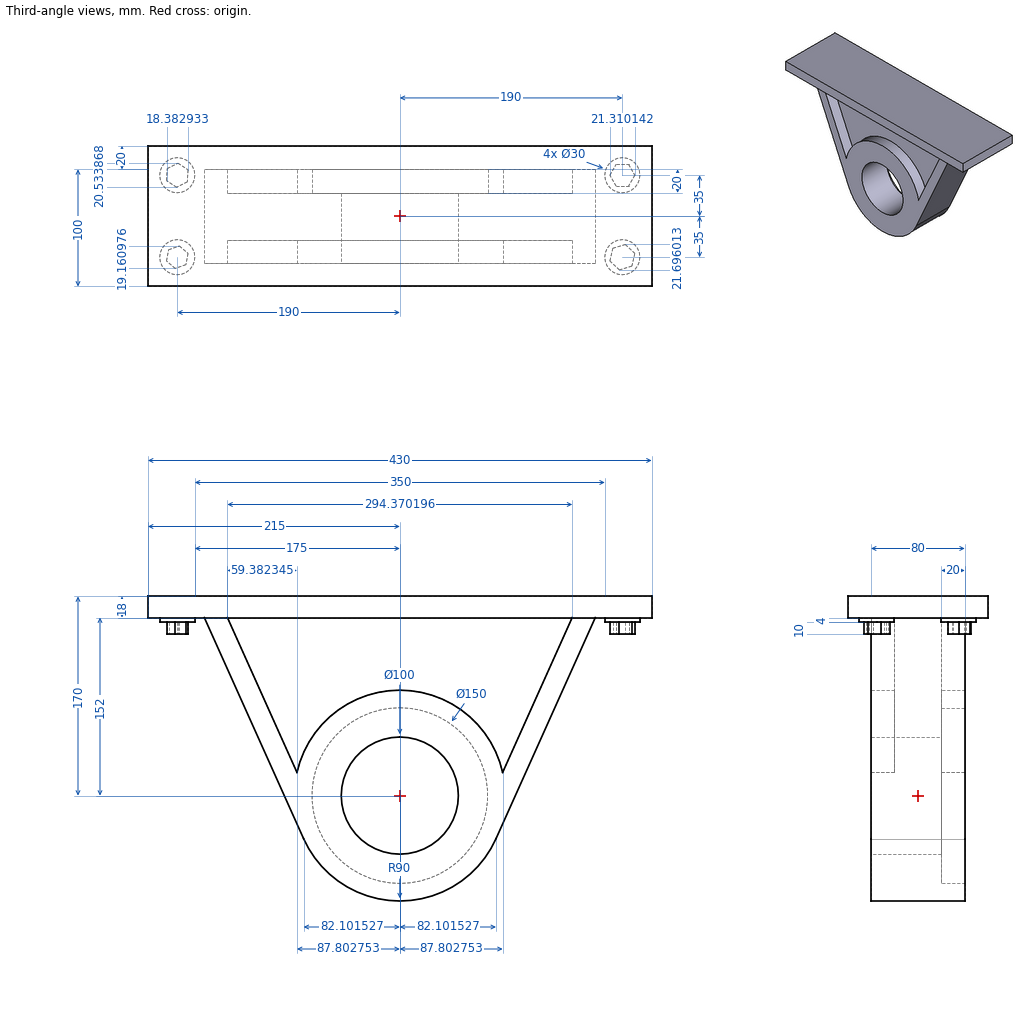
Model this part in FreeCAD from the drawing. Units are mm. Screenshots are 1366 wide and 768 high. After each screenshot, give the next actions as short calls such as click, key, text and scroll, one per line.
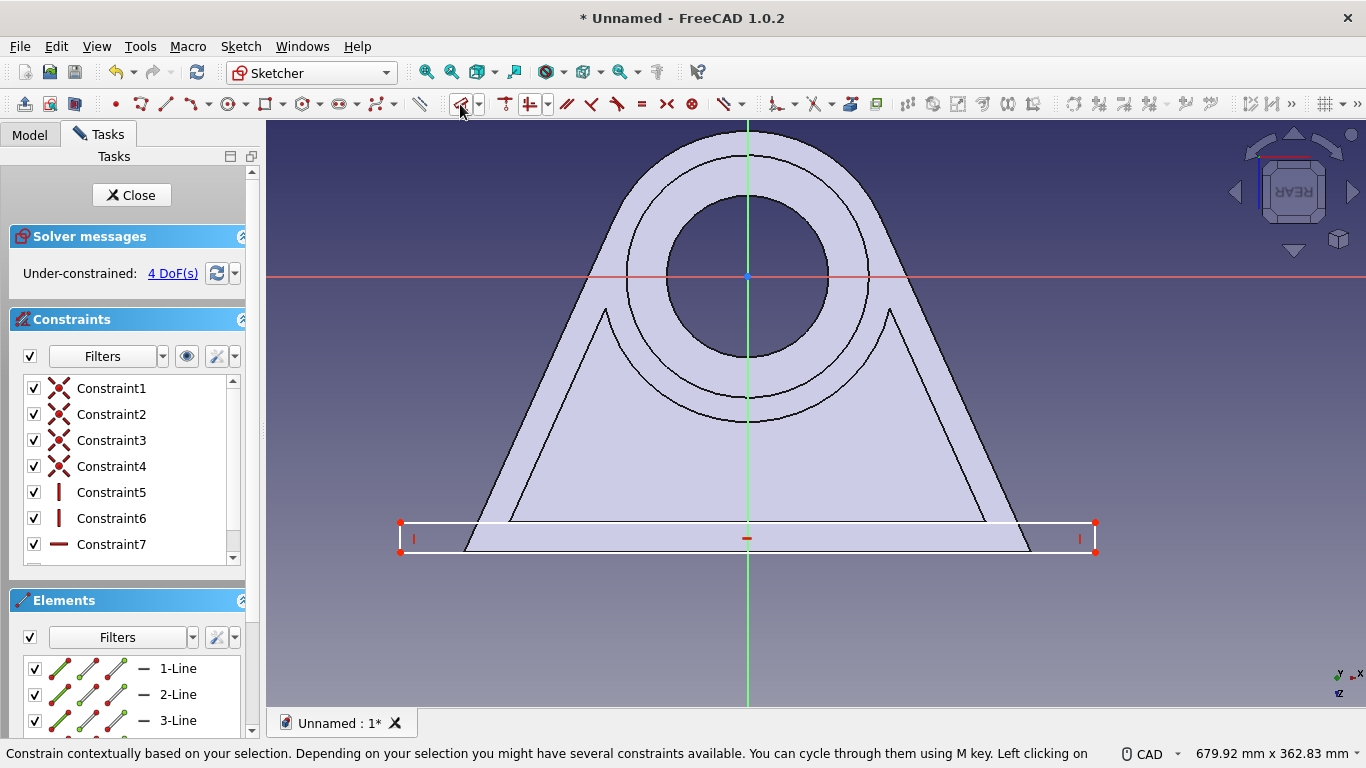
scroll(400, 535, up, 2)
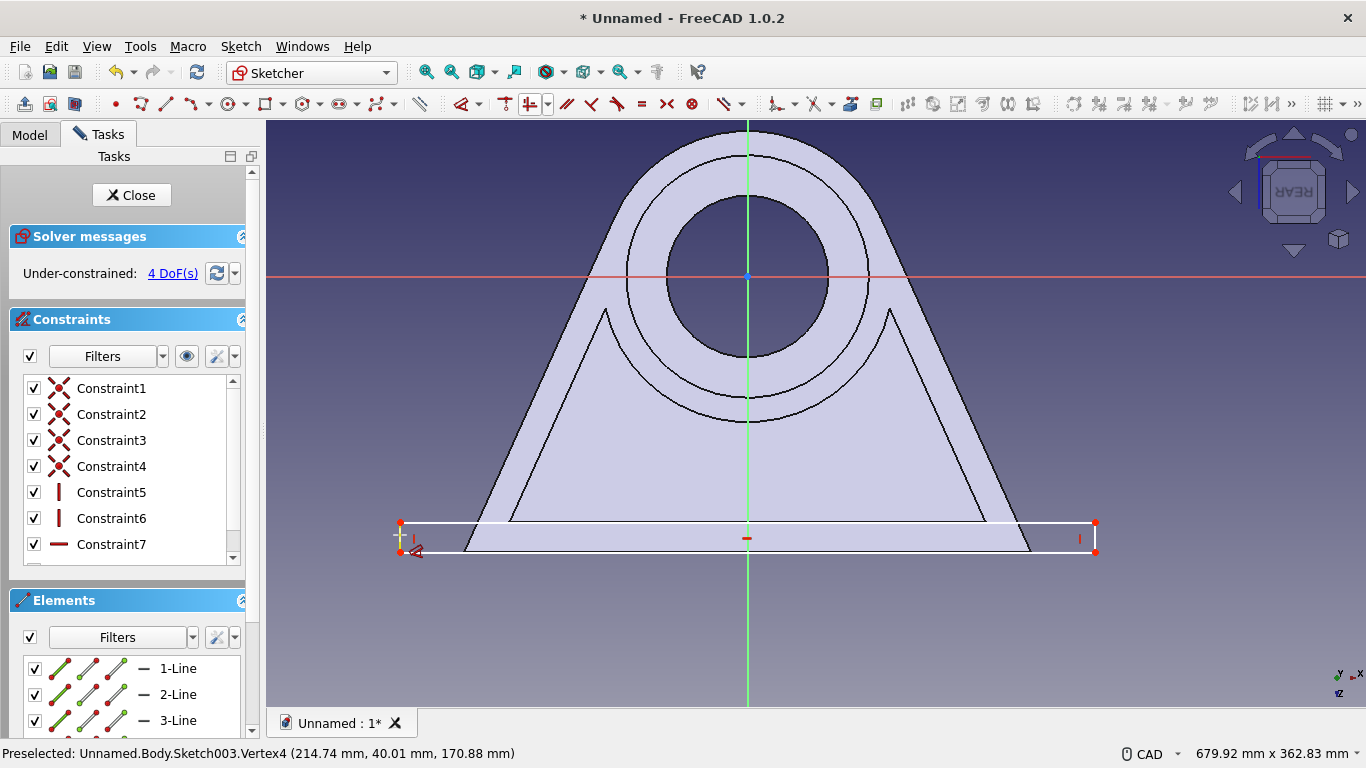
click(400, 535)
click(366, 539)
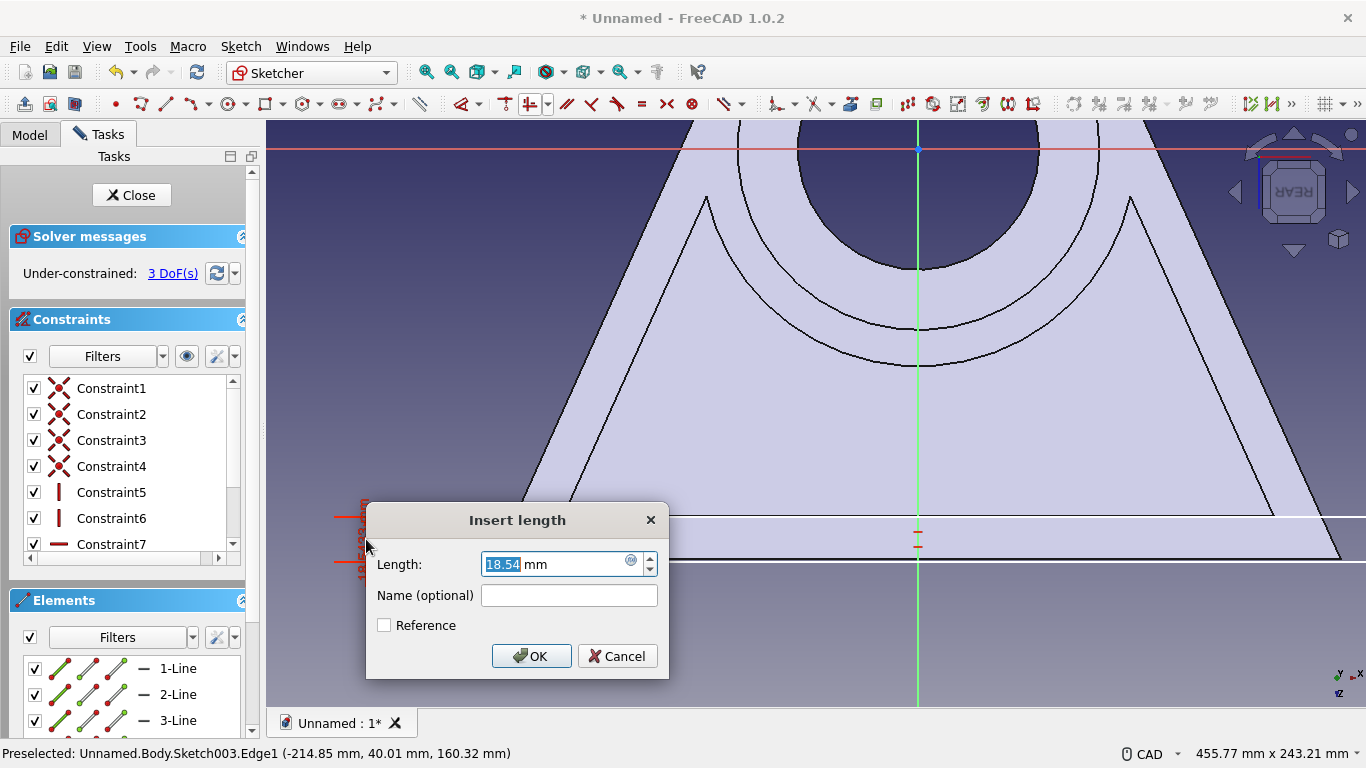
text(18)
key(Return)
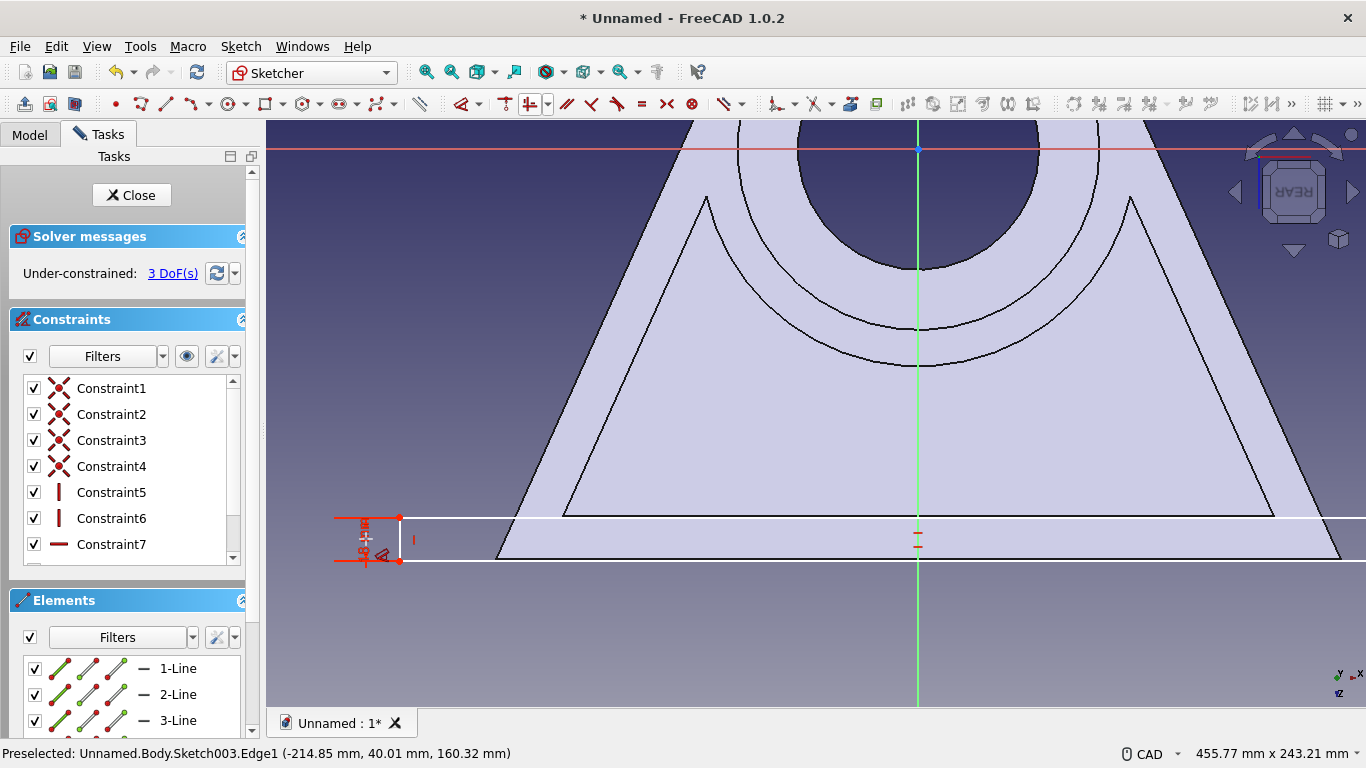
click(711, 561)
click(800, 595)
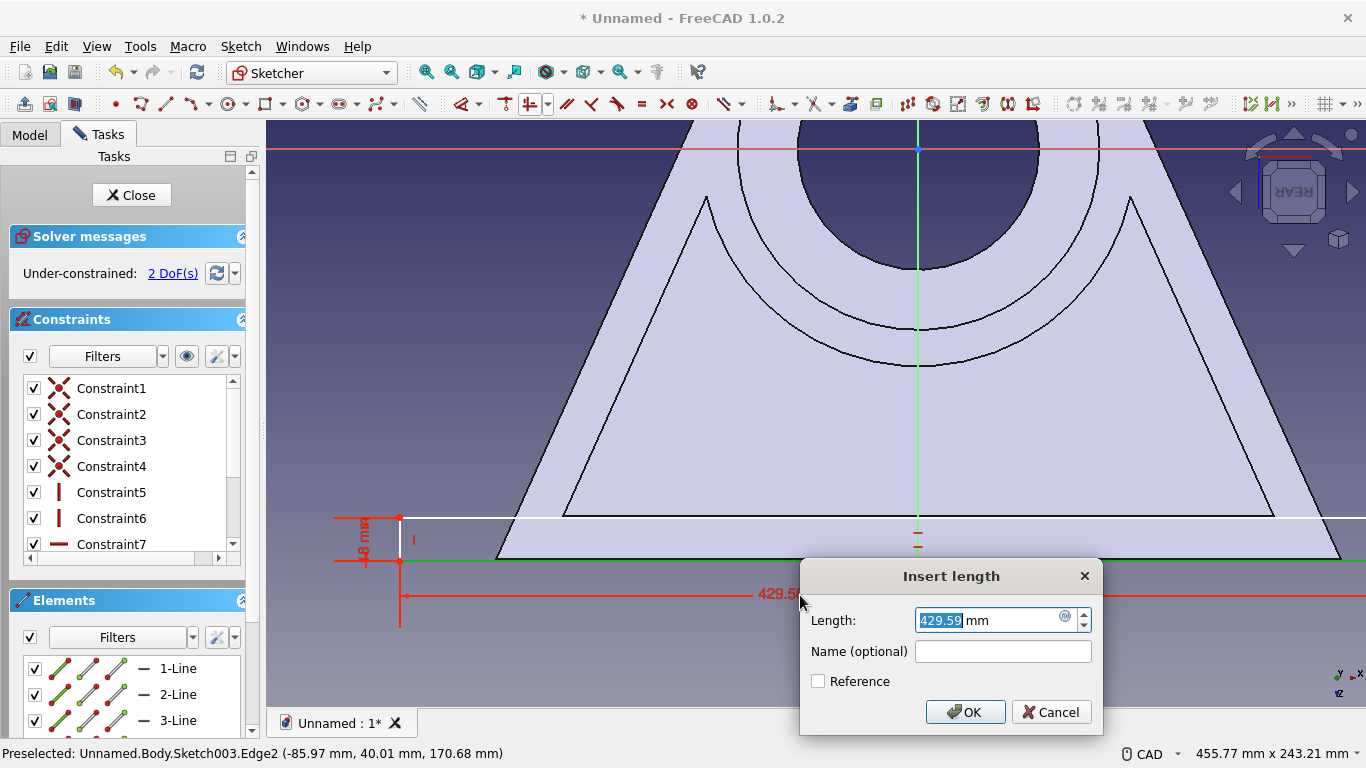
text(430)
key(Return)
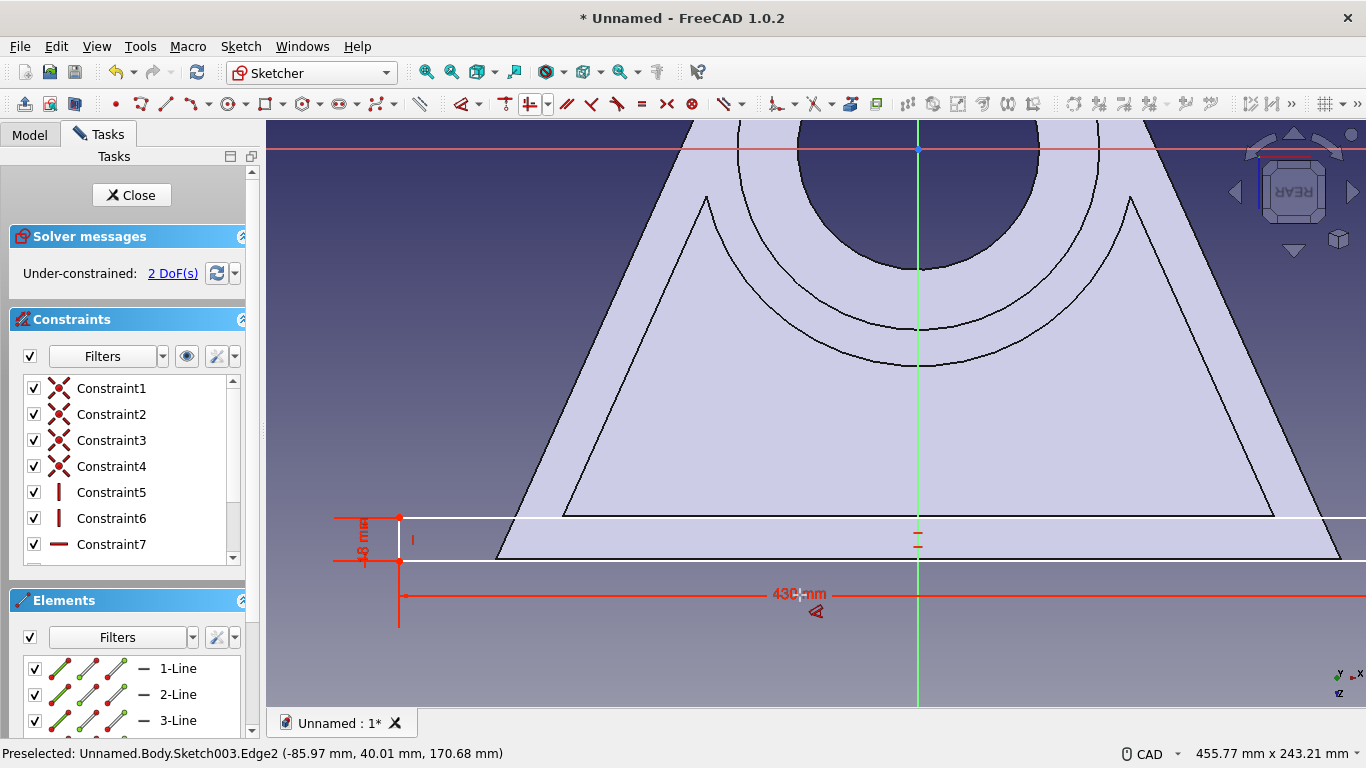
click(399, 518)
click(659, 576)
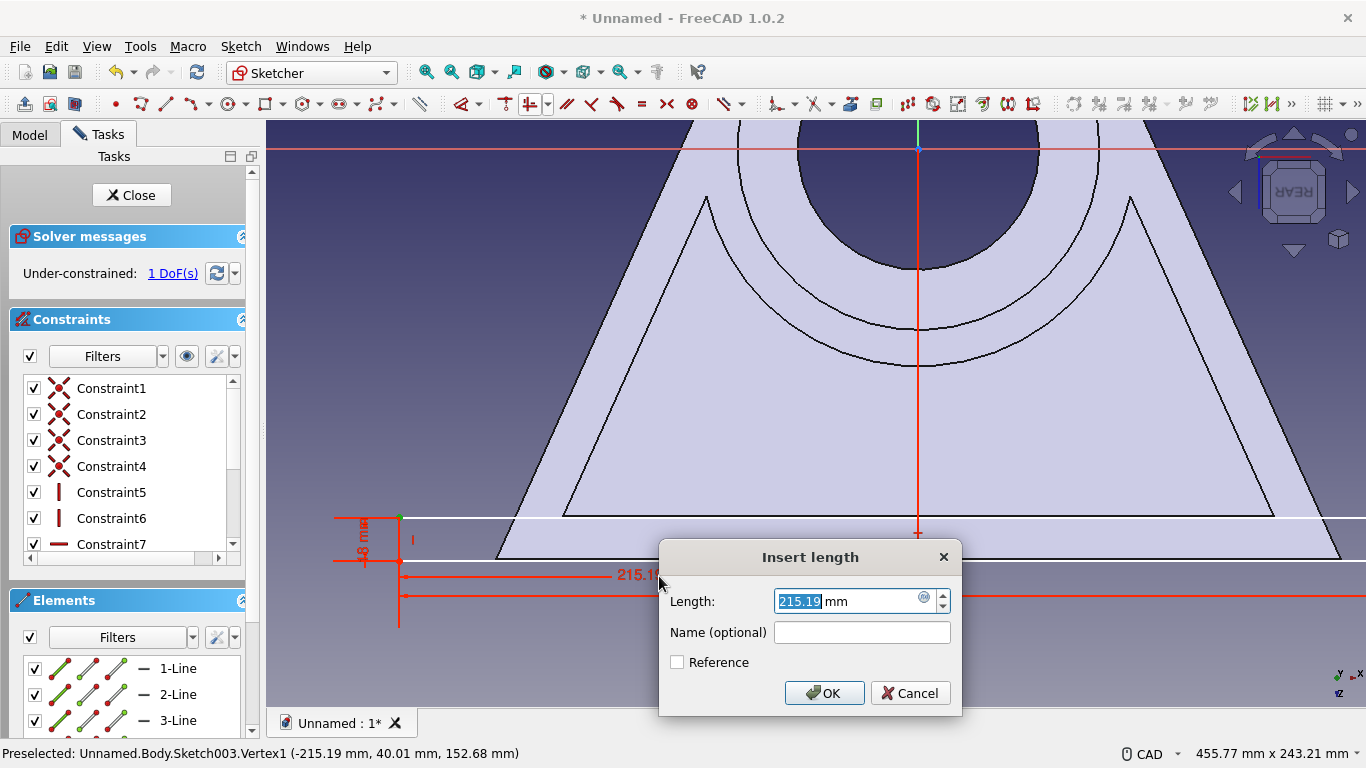
text(215)
key(Return)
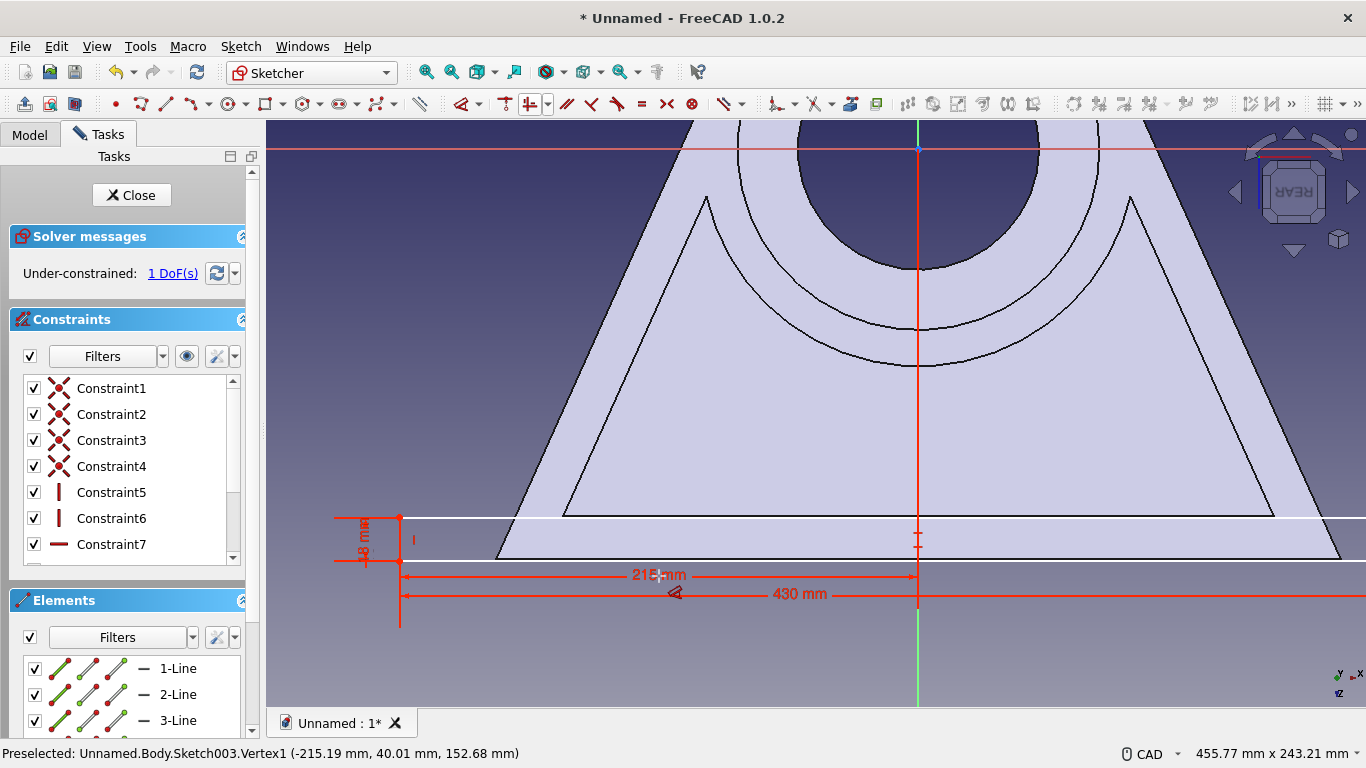
click(400, 518)
click(366, 333)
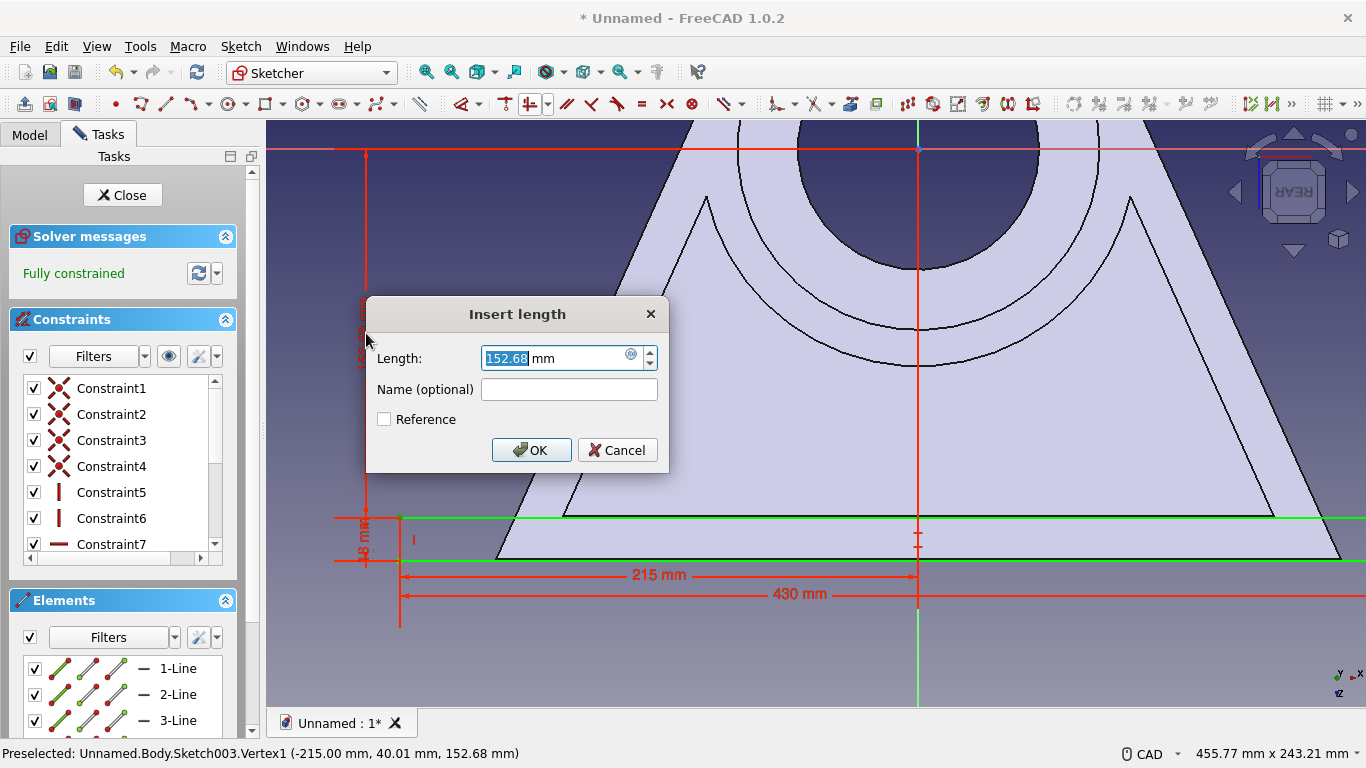
text(152)
key(Return)
key(Escape)